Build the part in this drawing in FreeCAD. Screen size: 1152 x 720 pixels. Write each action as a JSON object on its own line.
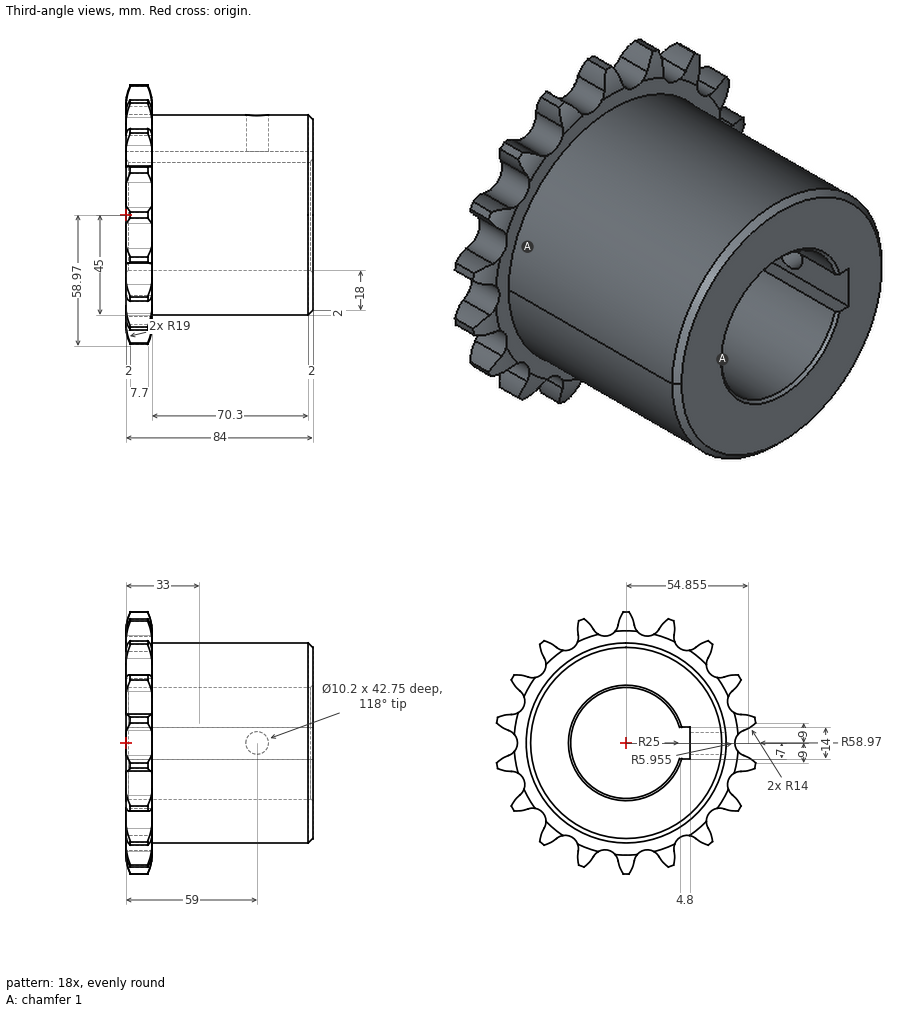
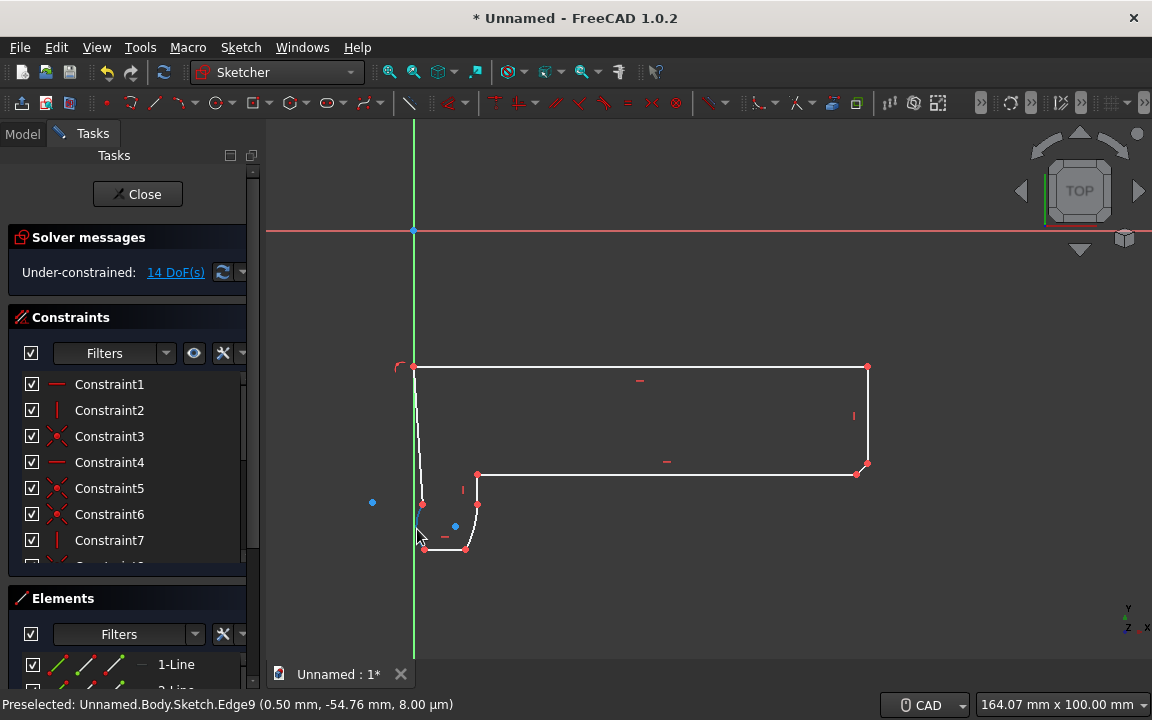
{"action": "scroll", "coordinate": [477, 495], "scroll_direction": "up", "scroll_amount": 3}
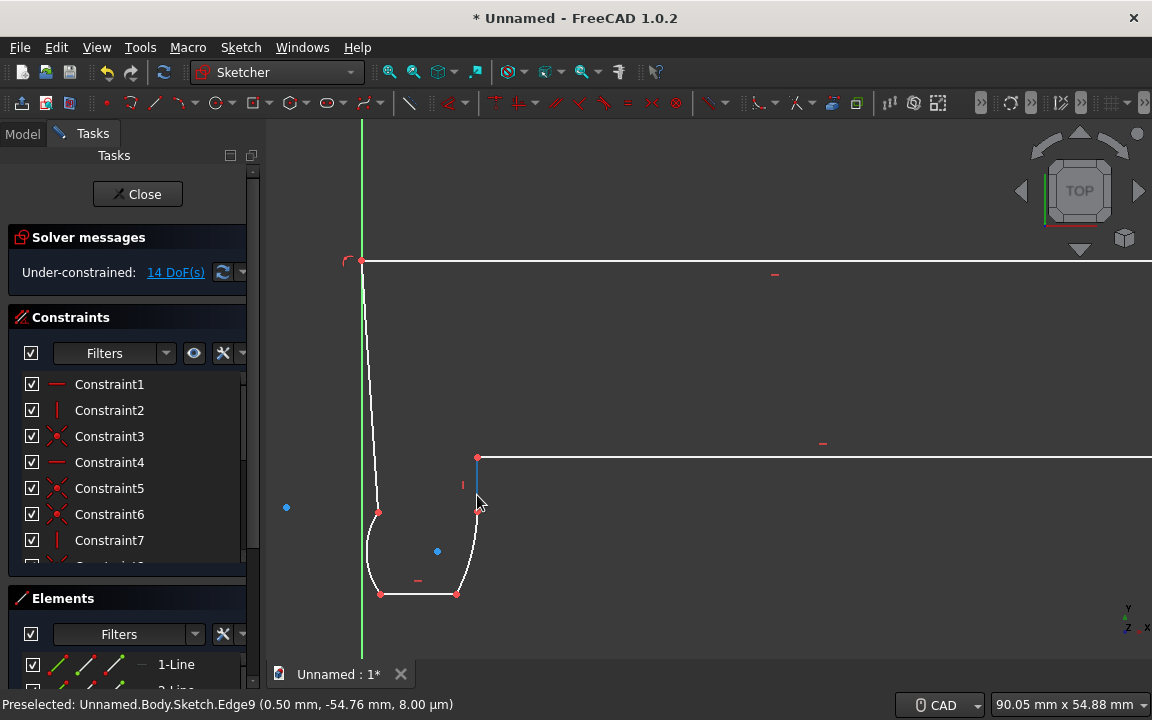
{"action": "left_click", "coordinate": [477, 495]}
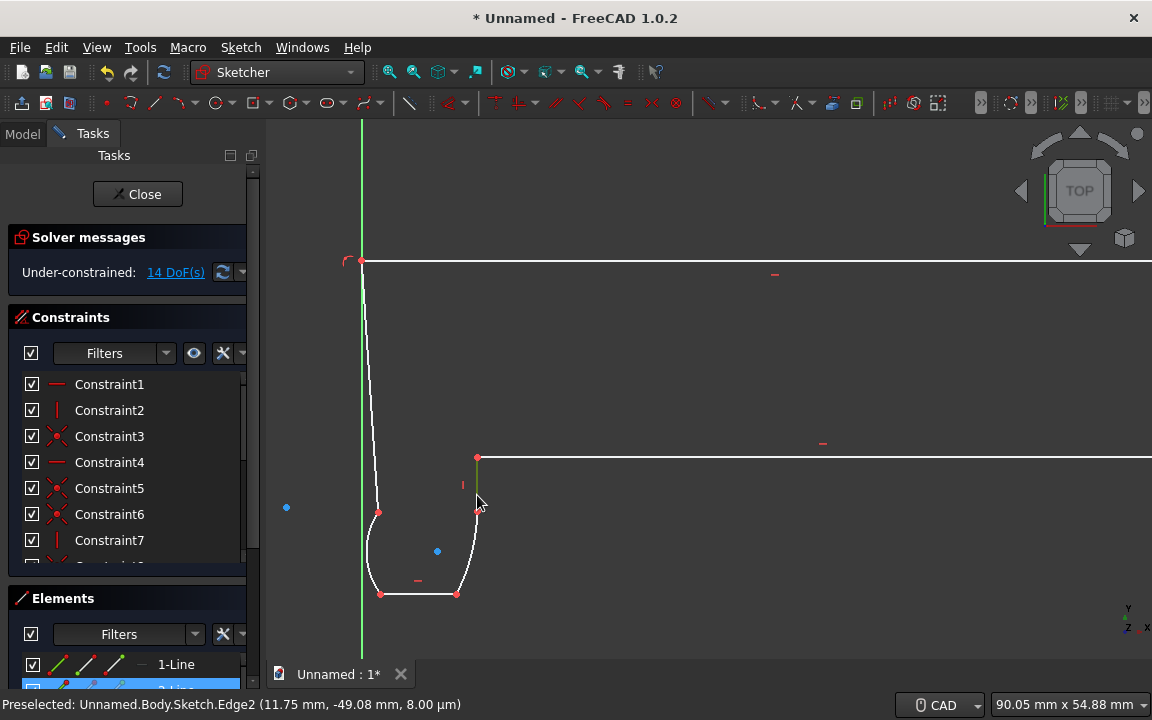
{"action": "left_click", "coordinate": [467, 570]}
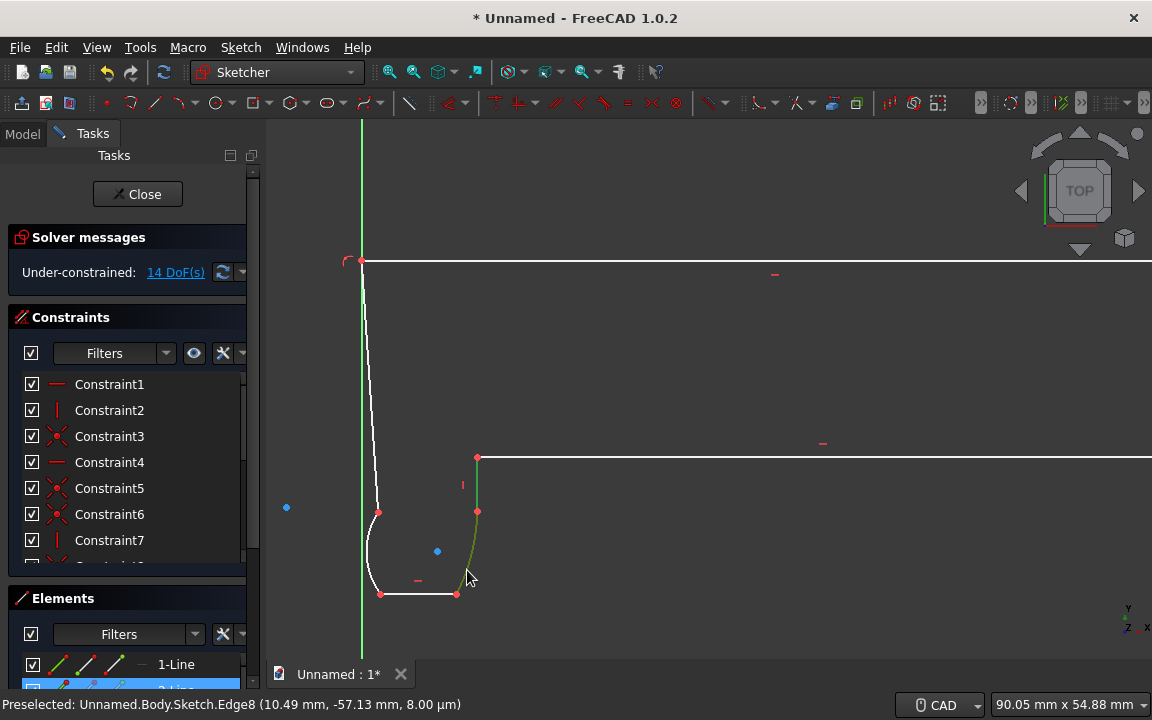
{"action": "key", "text": "t"}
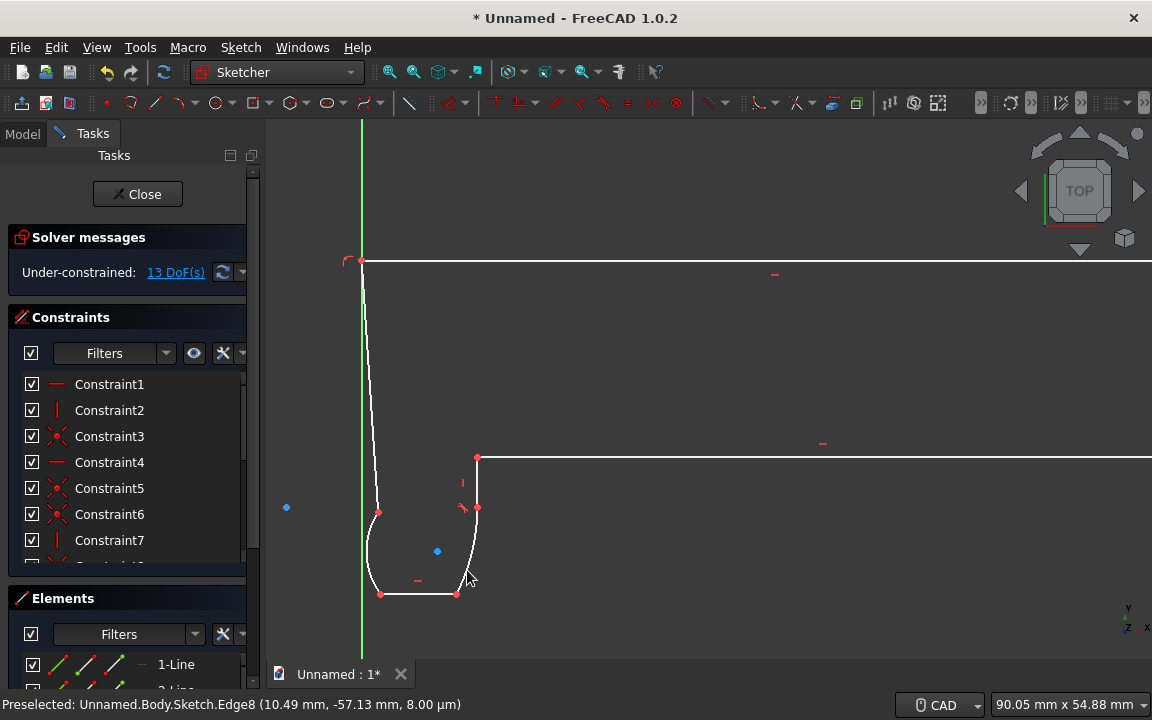
{"action": "left_click", "coordinate": [373, 437]}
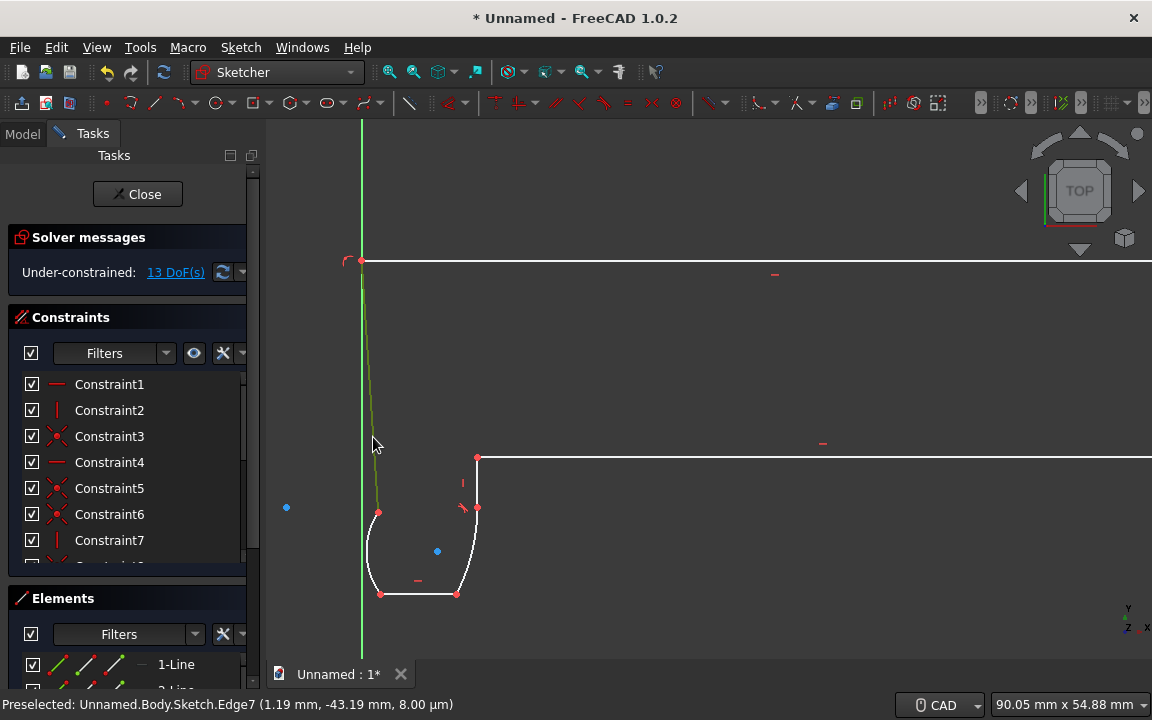
{"action": "scroll", "coordinate": [372, 579], "scroll_direction": "up", "scroll_amount": 2}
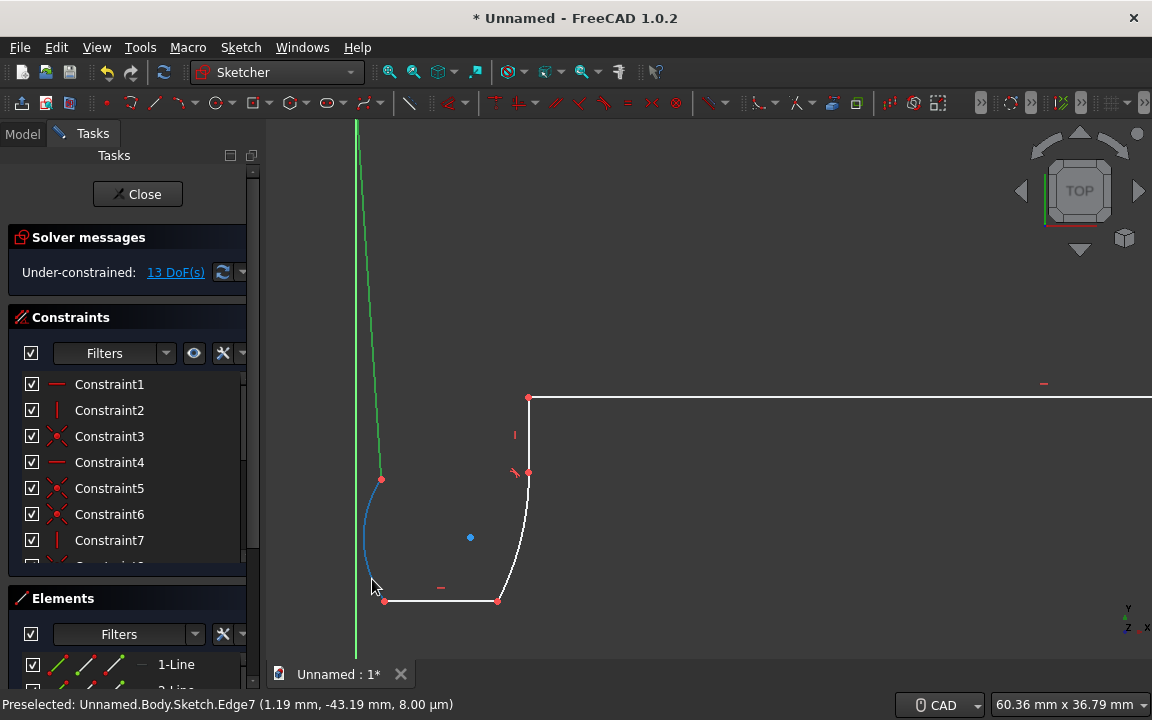
{"action": "left_click", "coordinate": [372, 579]}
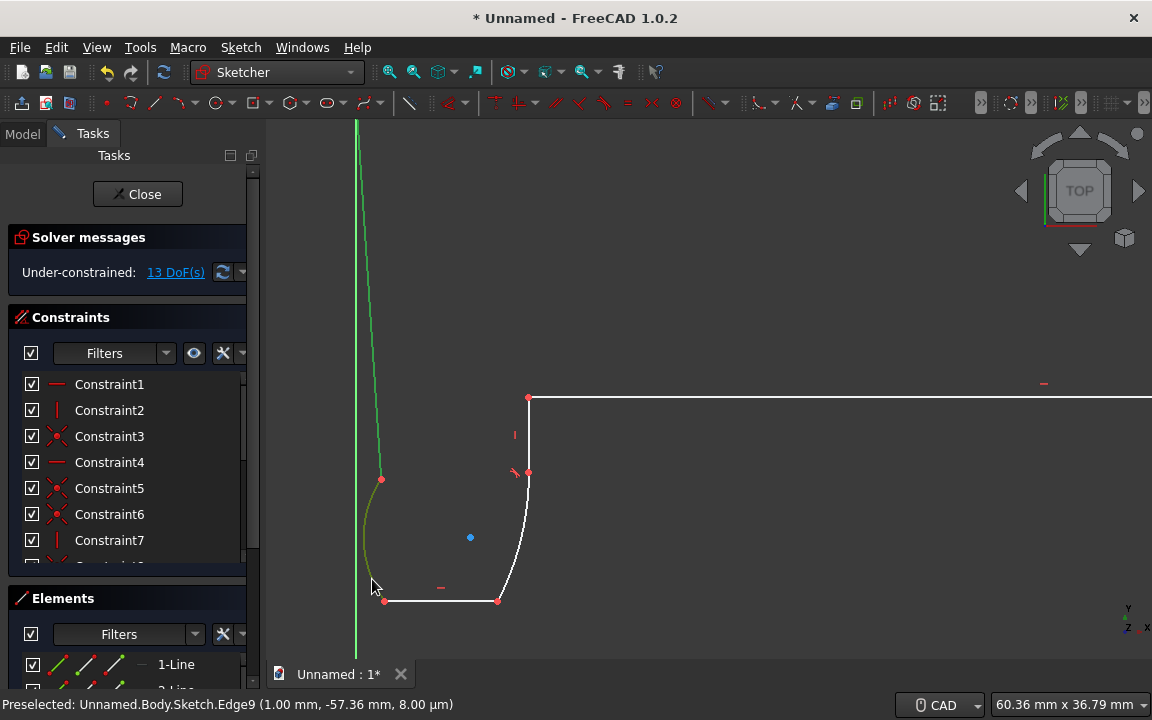
{"action": "key", "text": "t"}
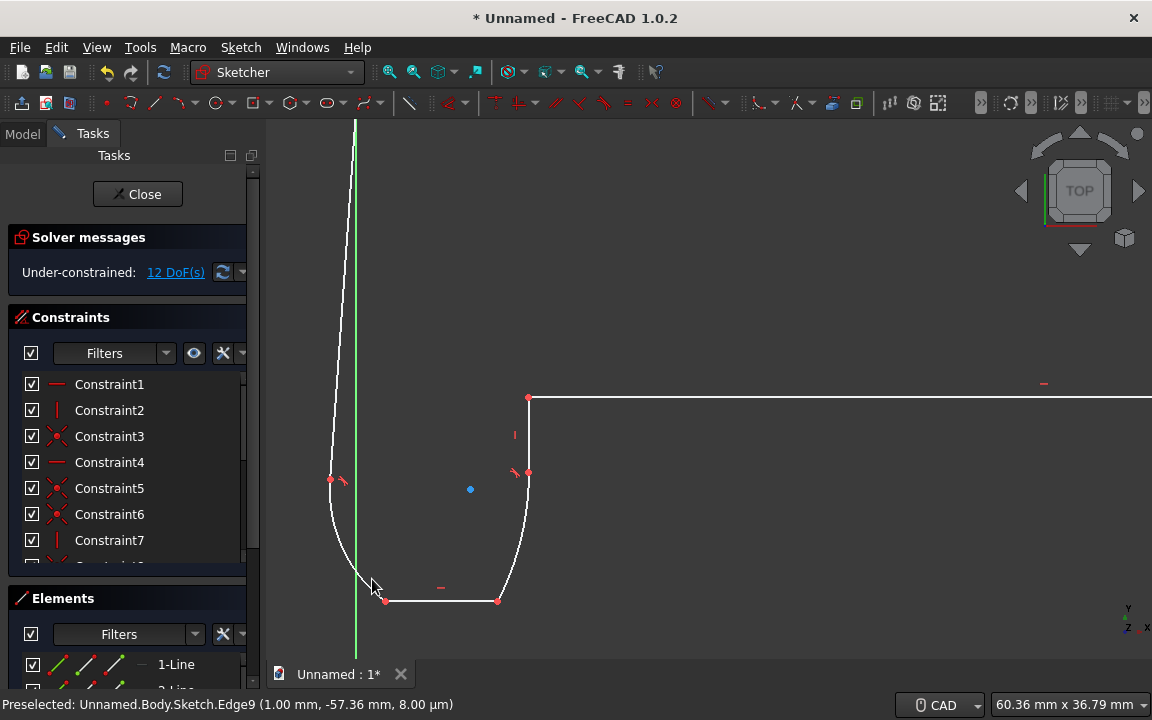
{"action": "left_click", "coordinate": [338, 367]}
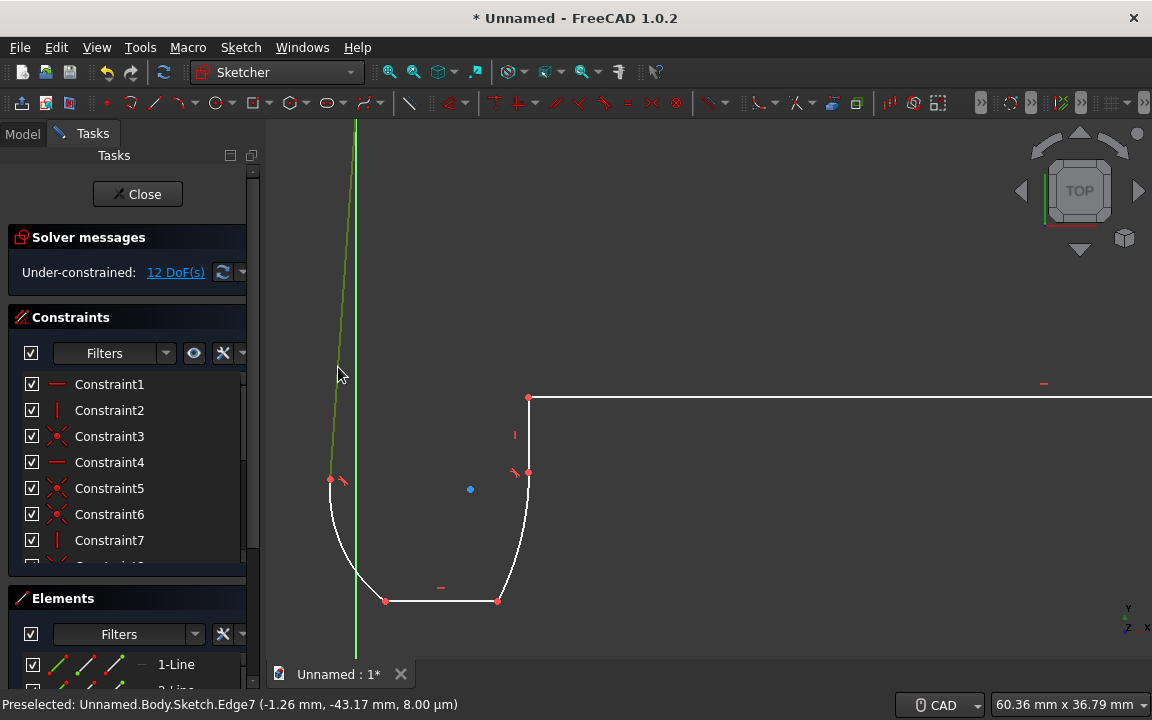
{"action": "key", "text": "v"}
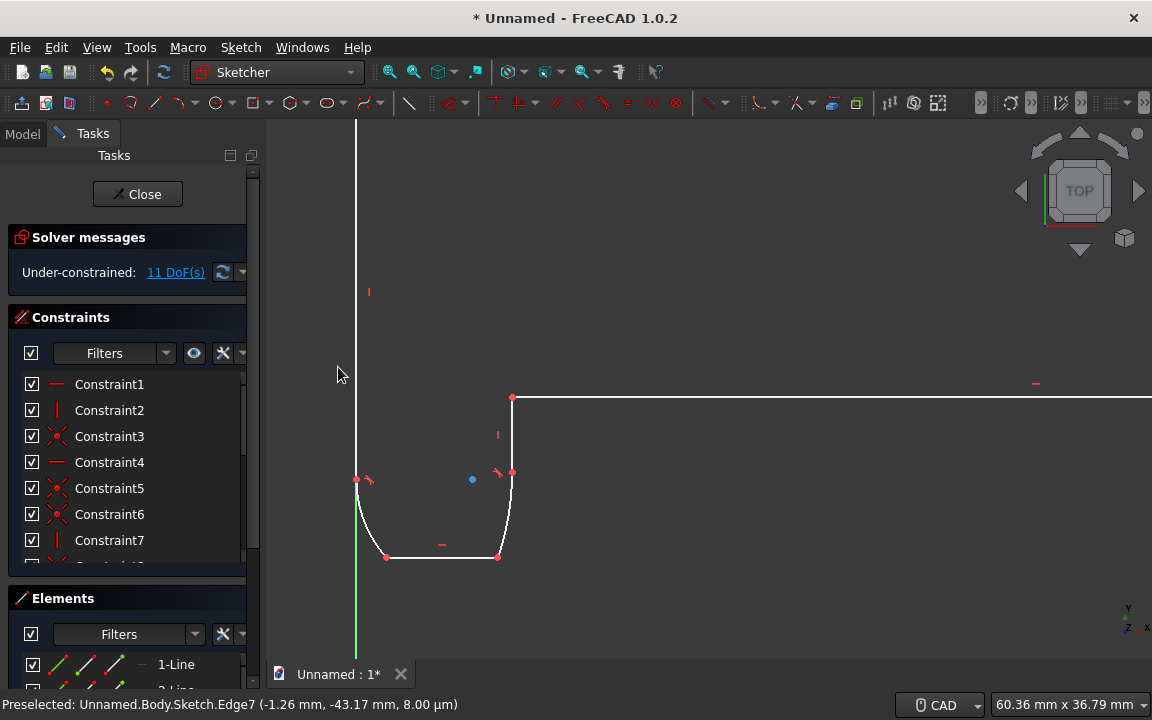
{"action": "left_click", "coordinate": [505, 533]}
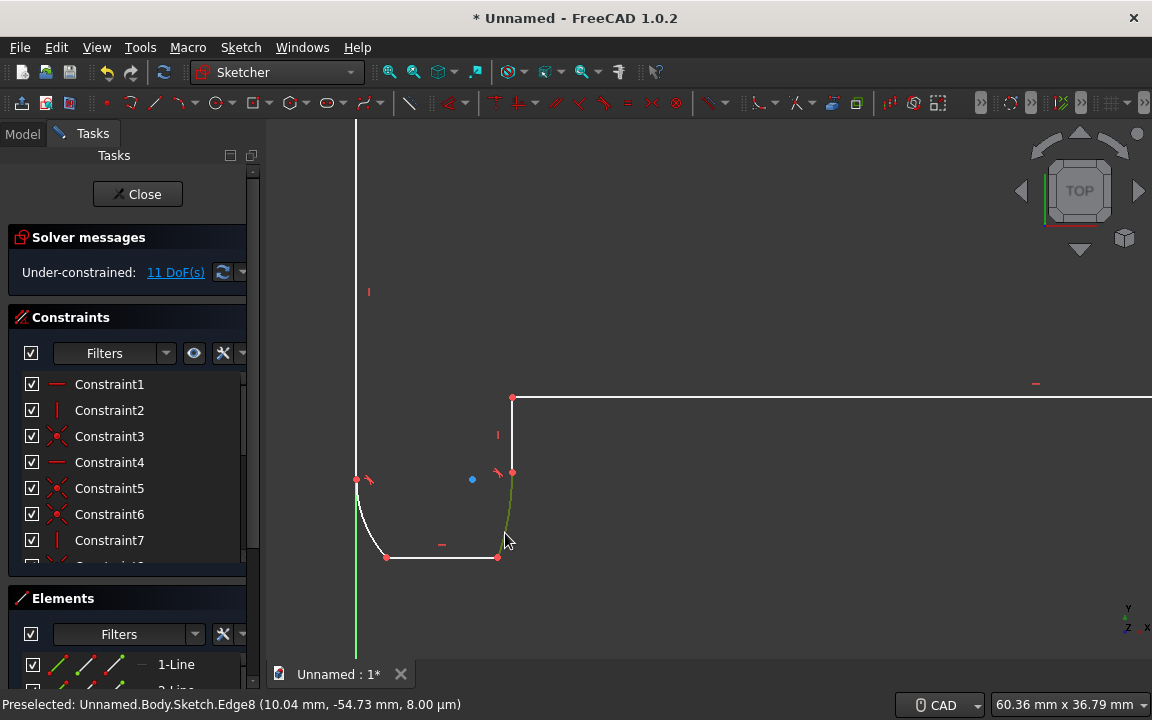
{"action": "left_click", "coordinate": [359, 505]}